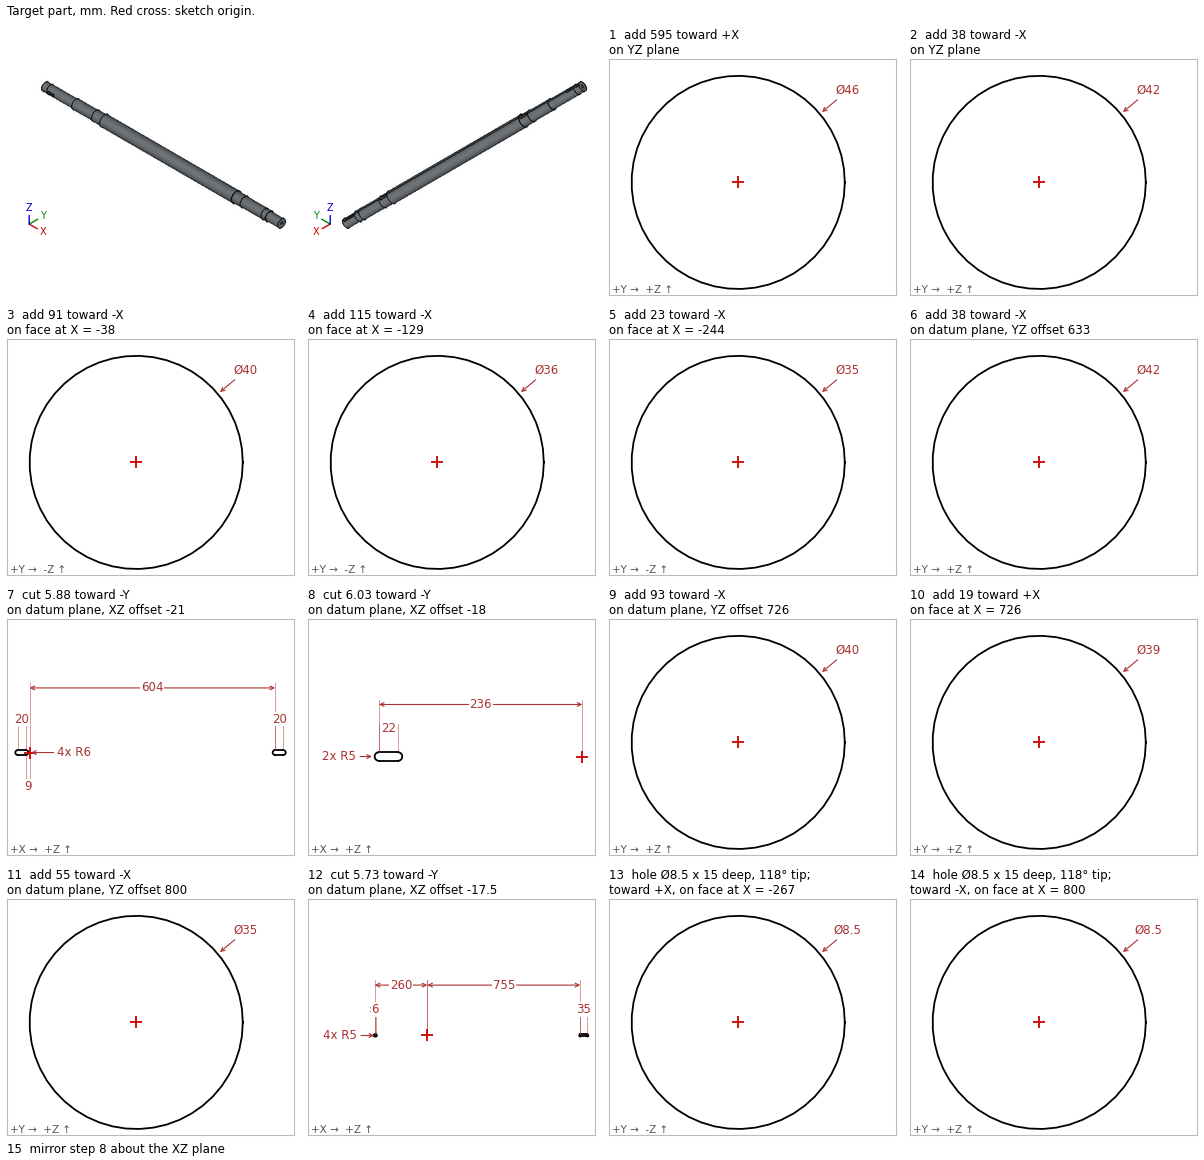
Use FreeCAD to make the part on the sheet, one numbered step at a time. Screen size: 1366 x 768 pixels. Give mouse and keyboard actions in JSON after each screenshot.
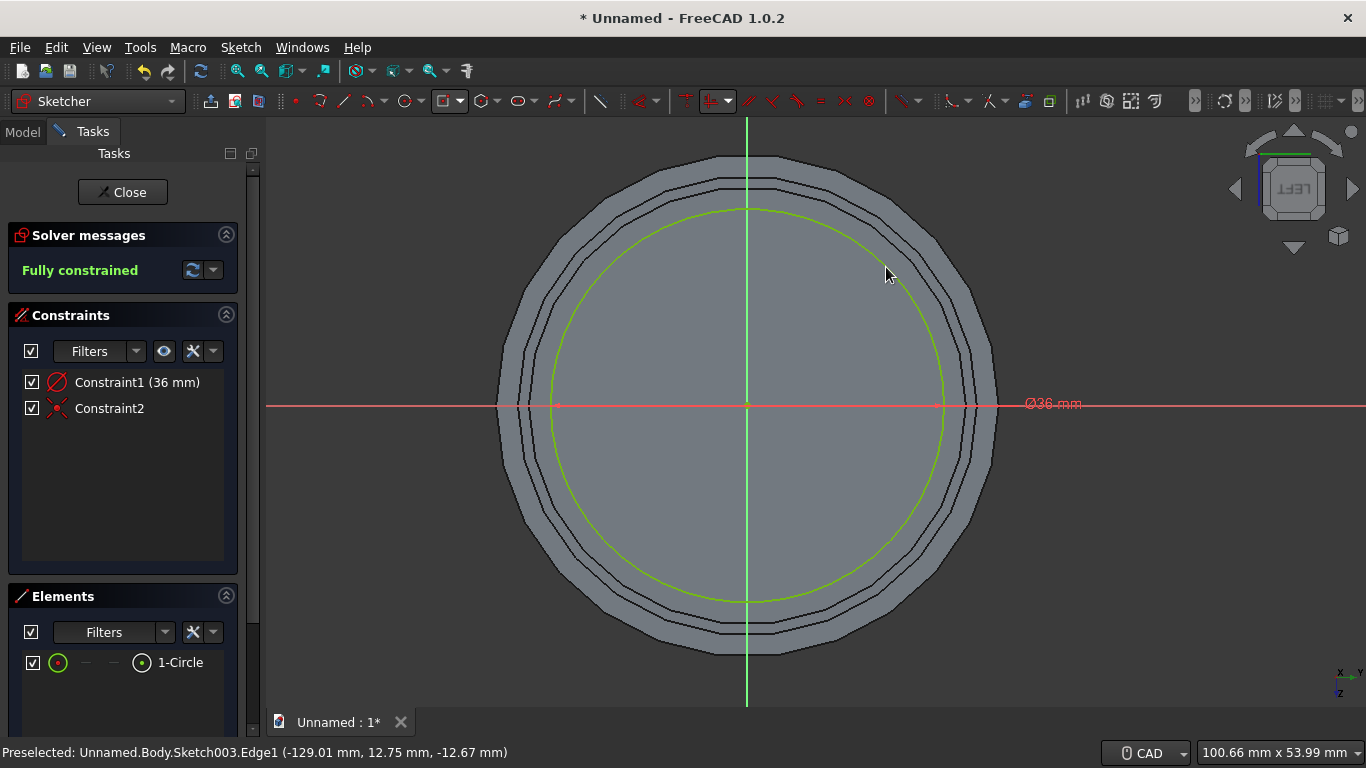
{"action": "left_click", "coordinate": [123, 192]}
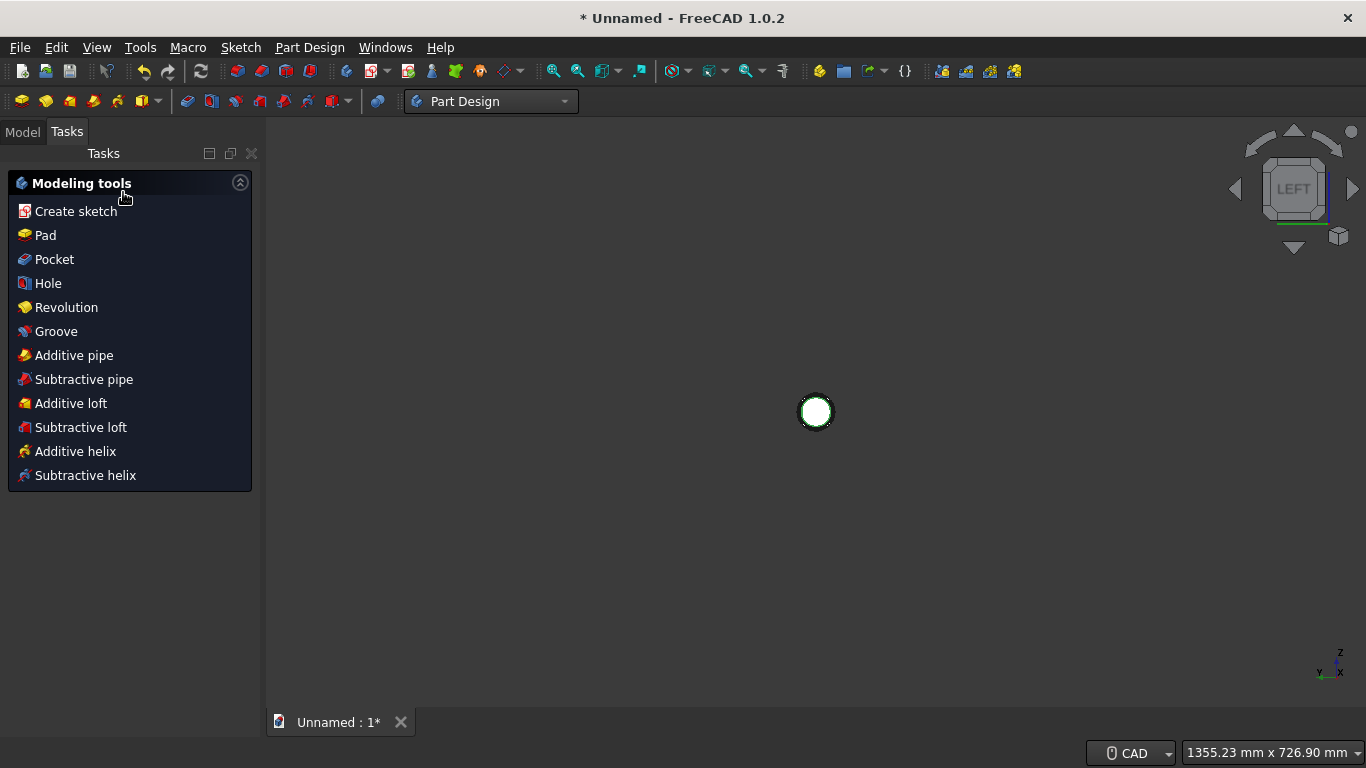
{"action": "left_click", "coordinate": [22, 102]}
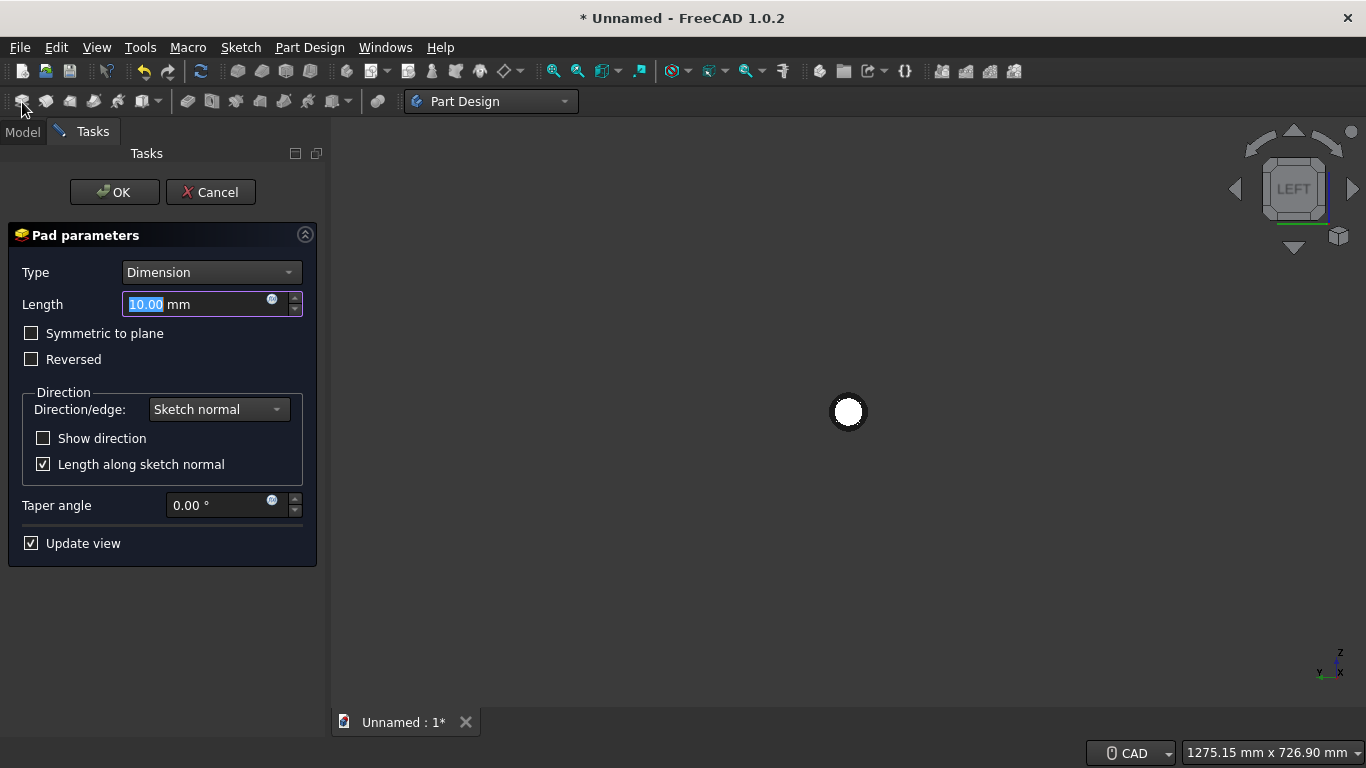
{"action": "type", "text": "115"}
{"action": "key", "text": "Tab"}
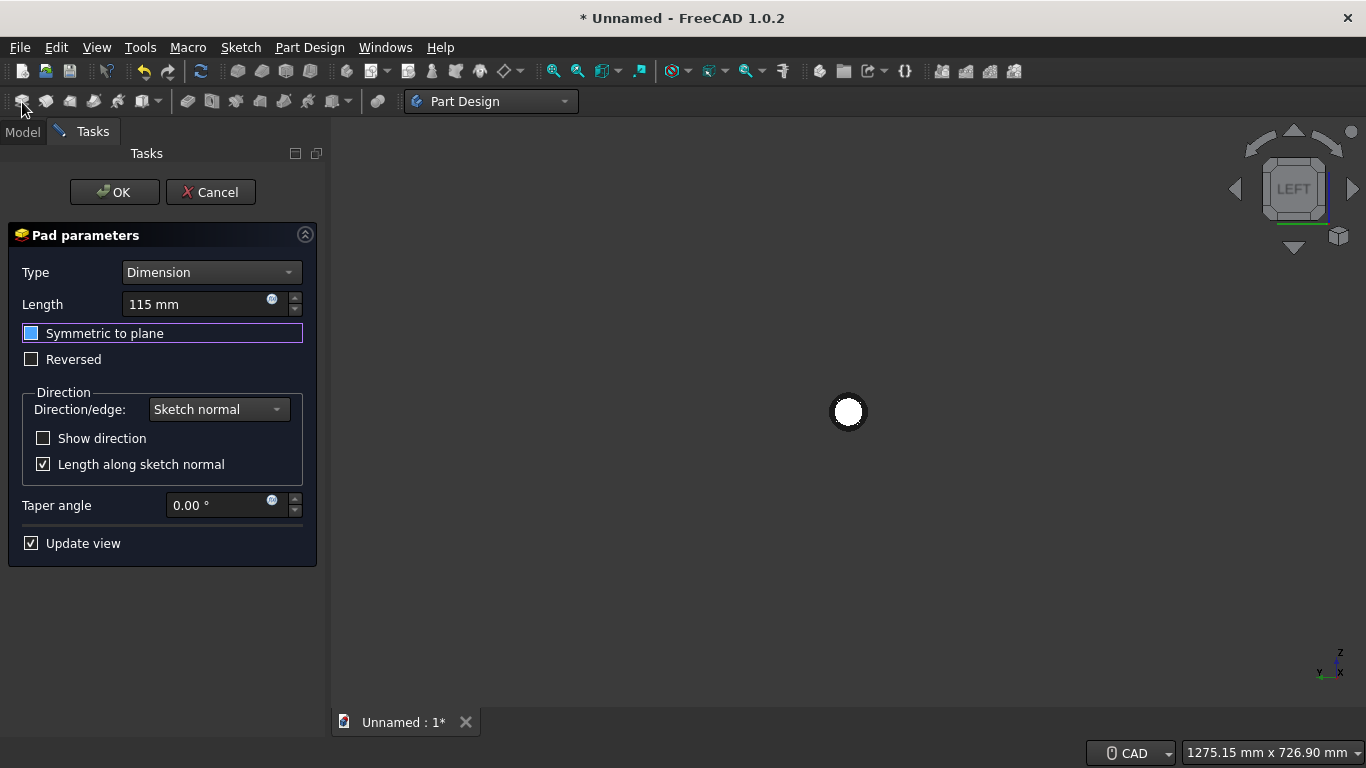
{"action": "left_click", "coordinate": [115, 192]}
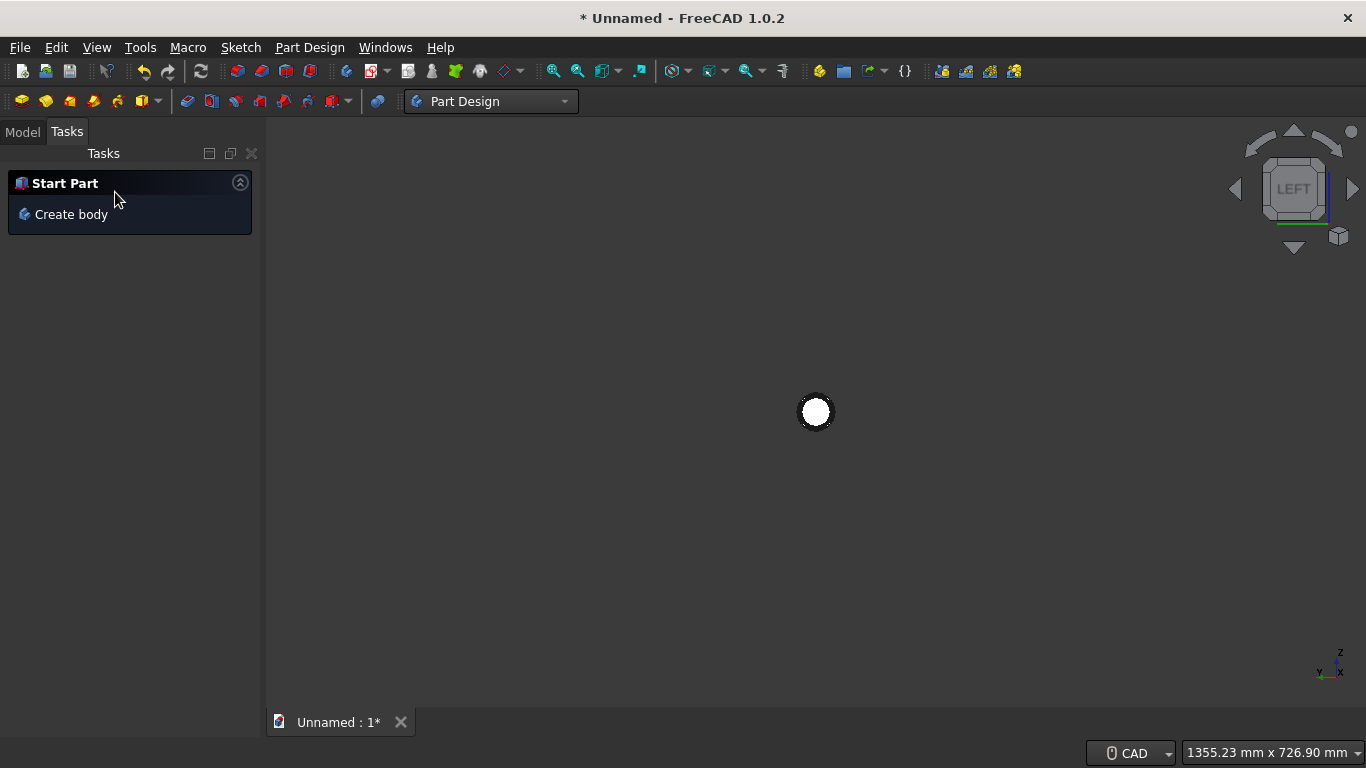
{"action": "left_click", "coordinate": [554, 72]}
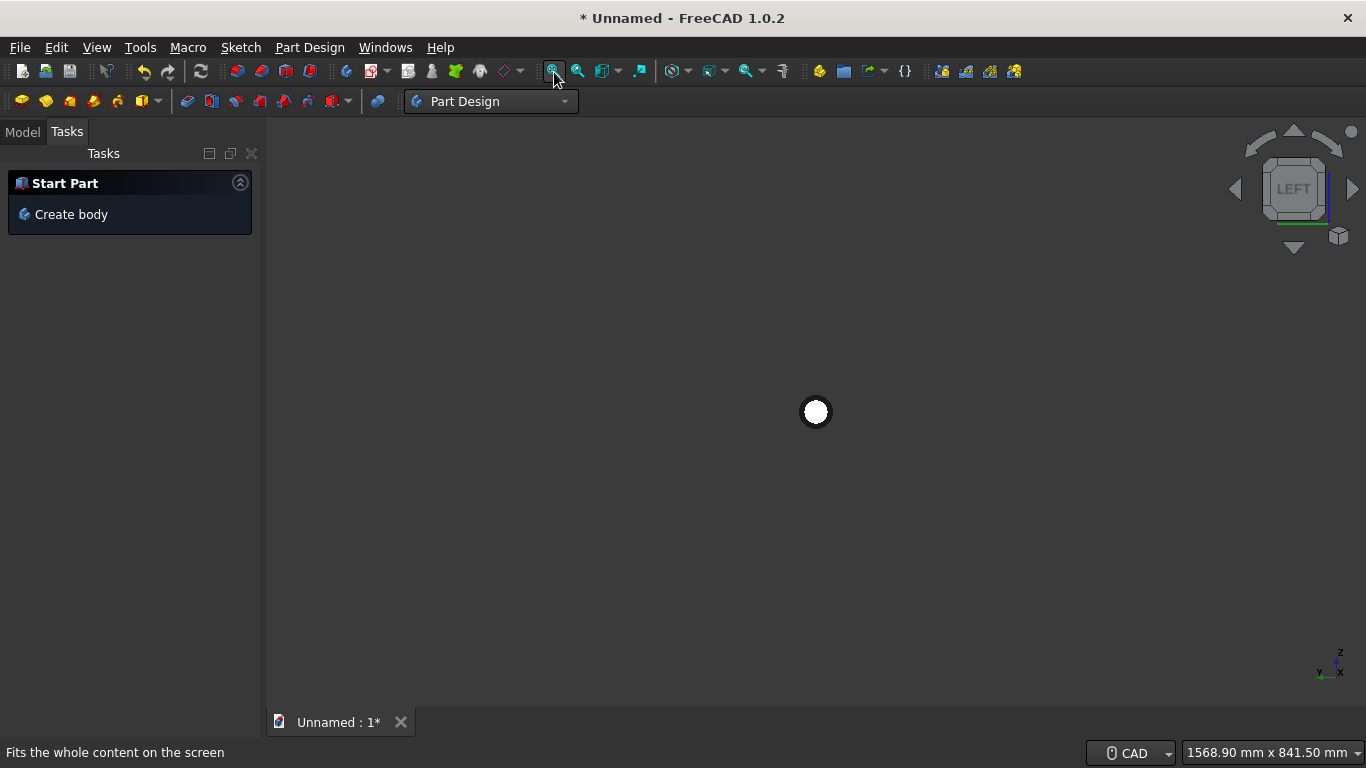
{"action": "left_click", "coordinate": [816, 411]}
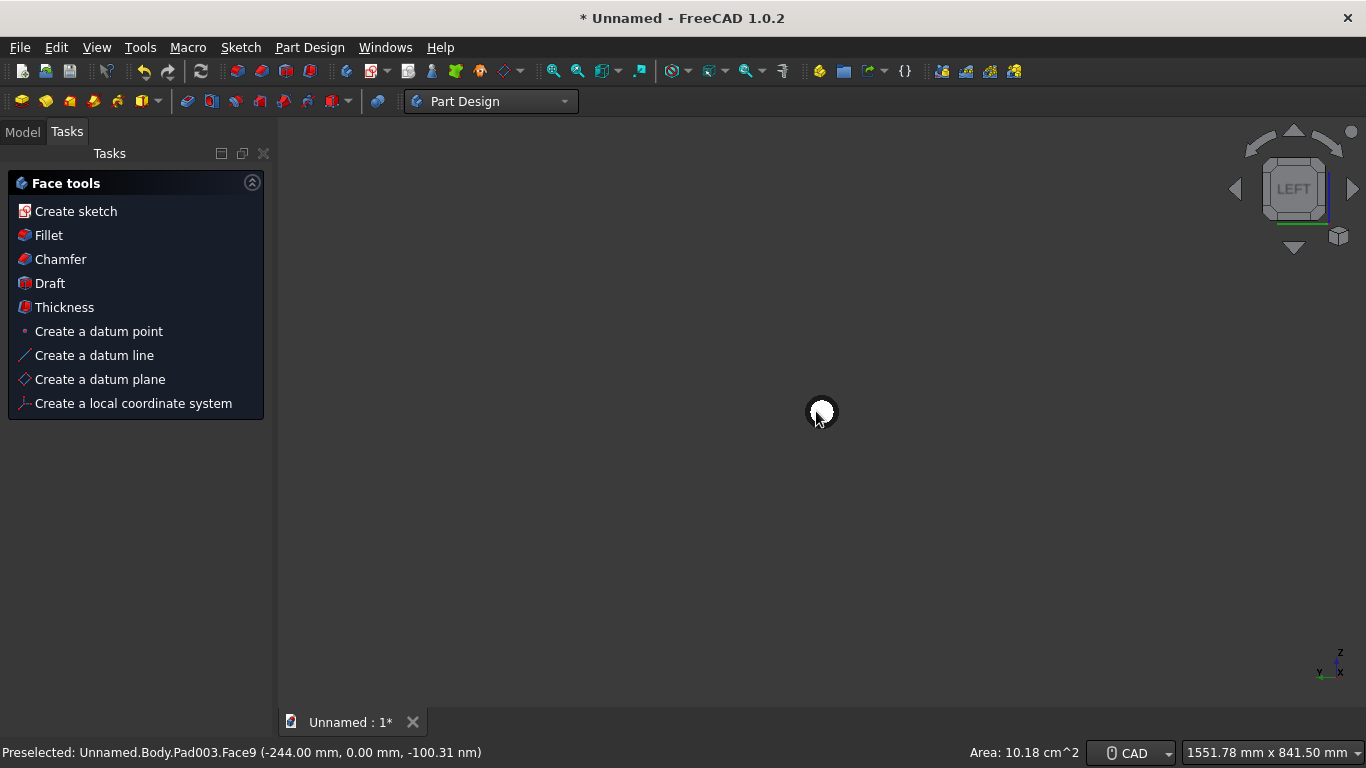
{"action": "left_click", "coordinate": [372, 72]}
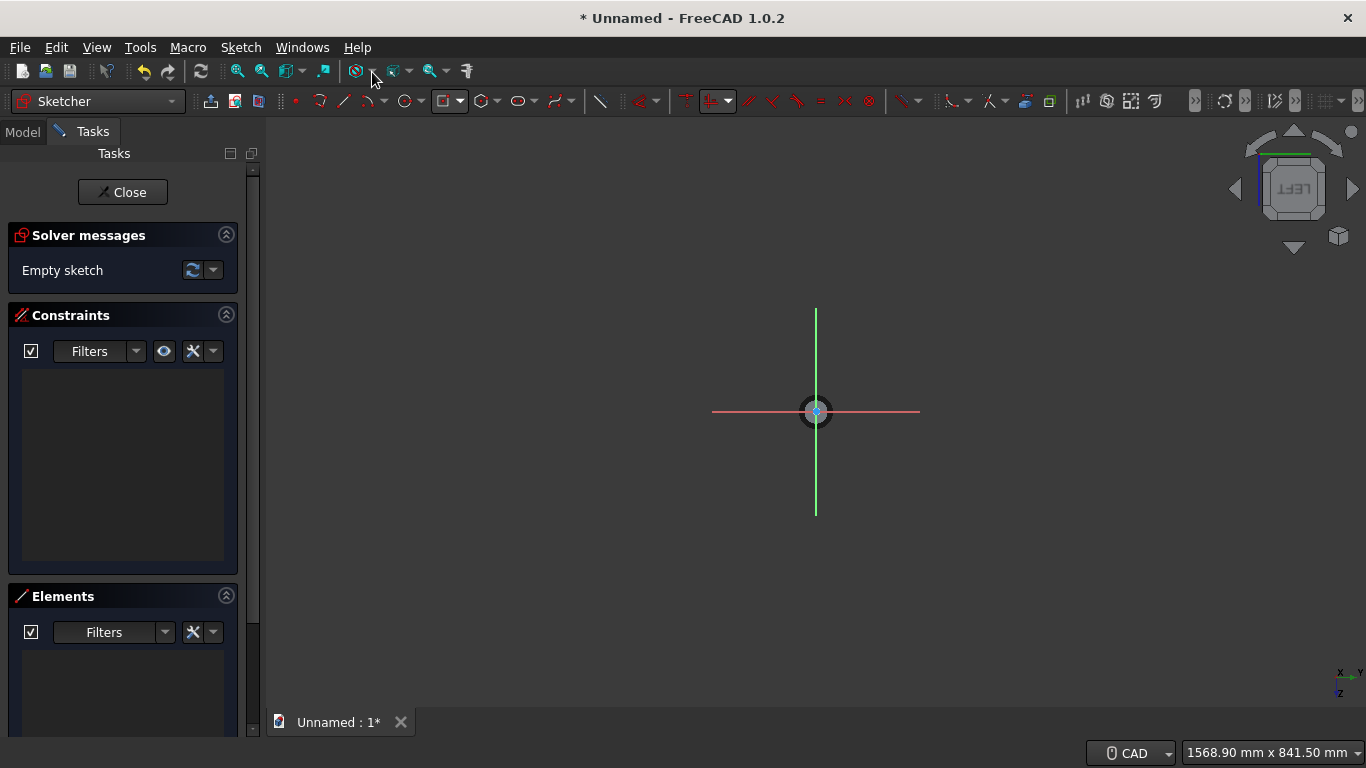
{"action": "scroll", "coordinate": [820, 412], "scroll_direction": "up", "scroll_amount": 14}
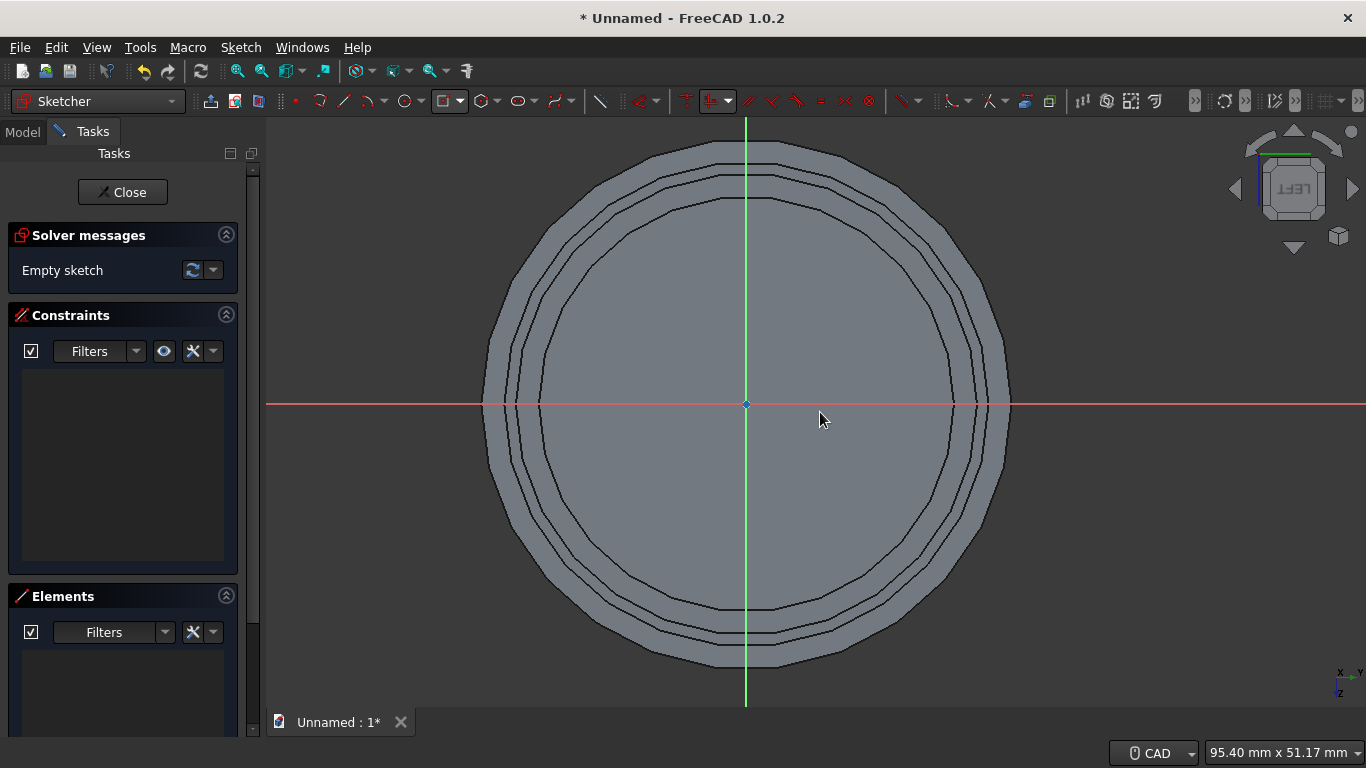
{"action": "key", "text": "g c"}